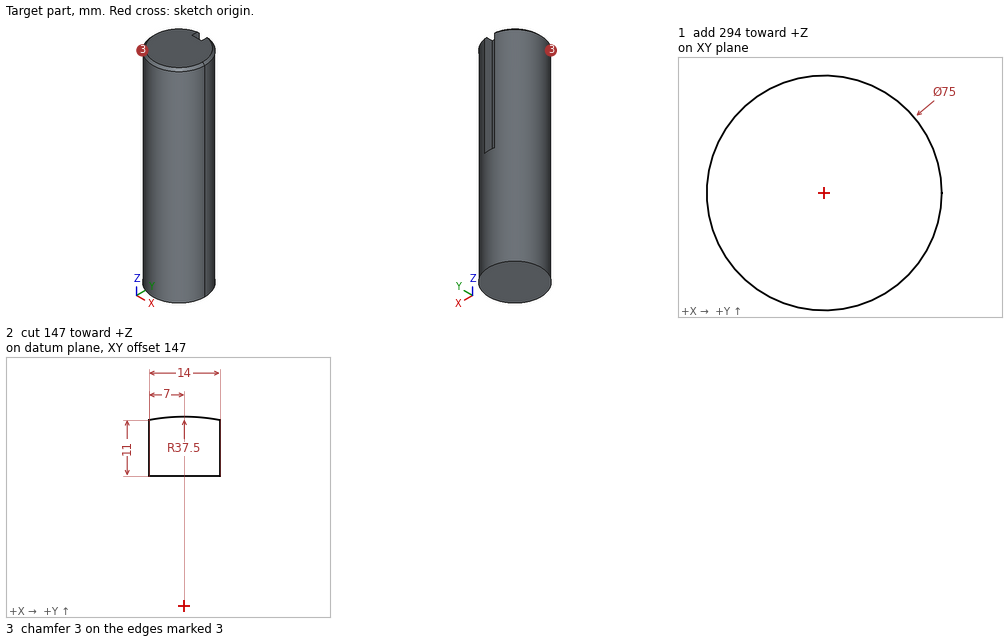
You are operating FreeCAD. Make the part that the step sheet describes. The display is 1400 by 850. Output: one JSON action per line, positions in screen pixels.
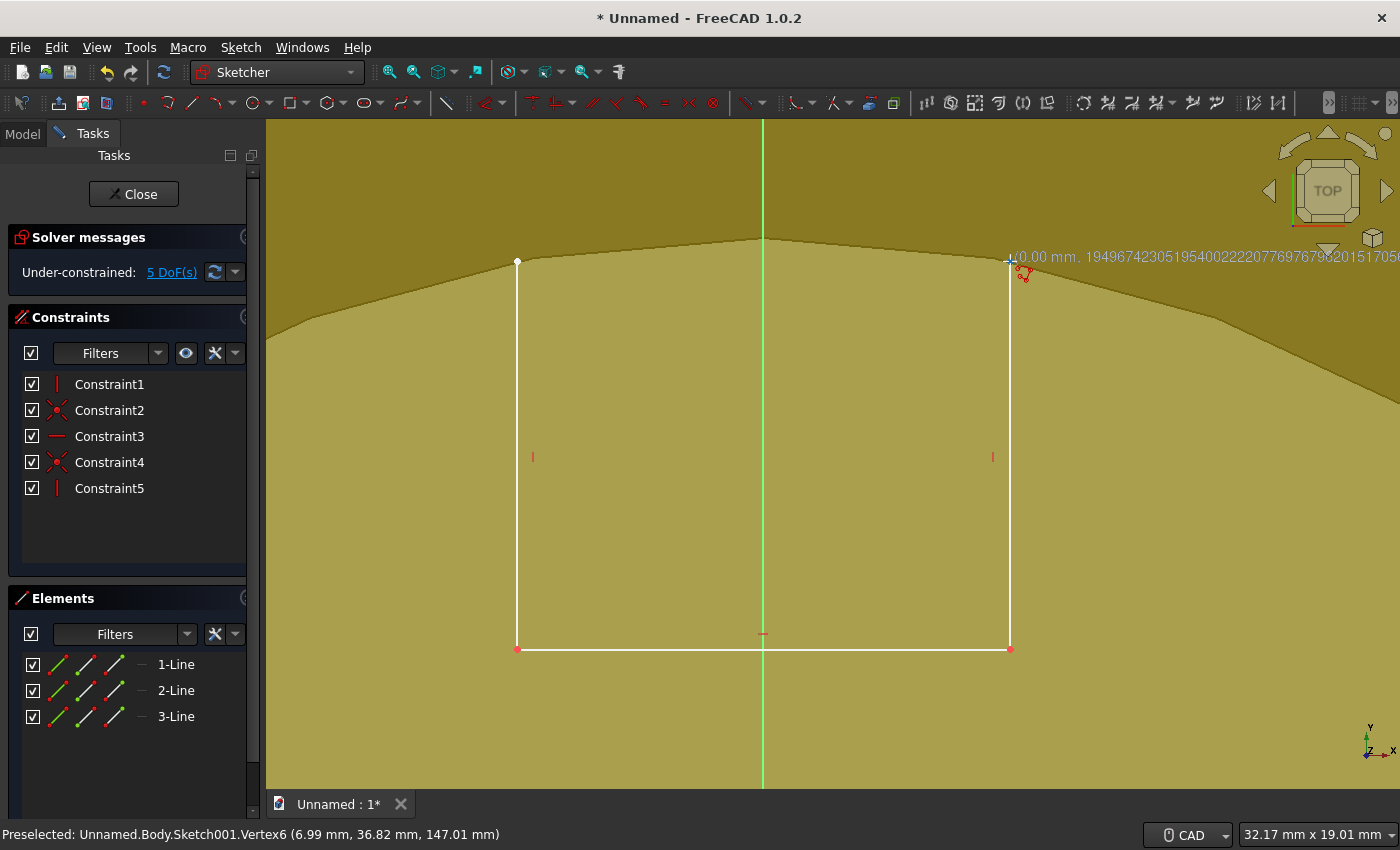
{"action": "left_click", "coordinate": [216, 104]}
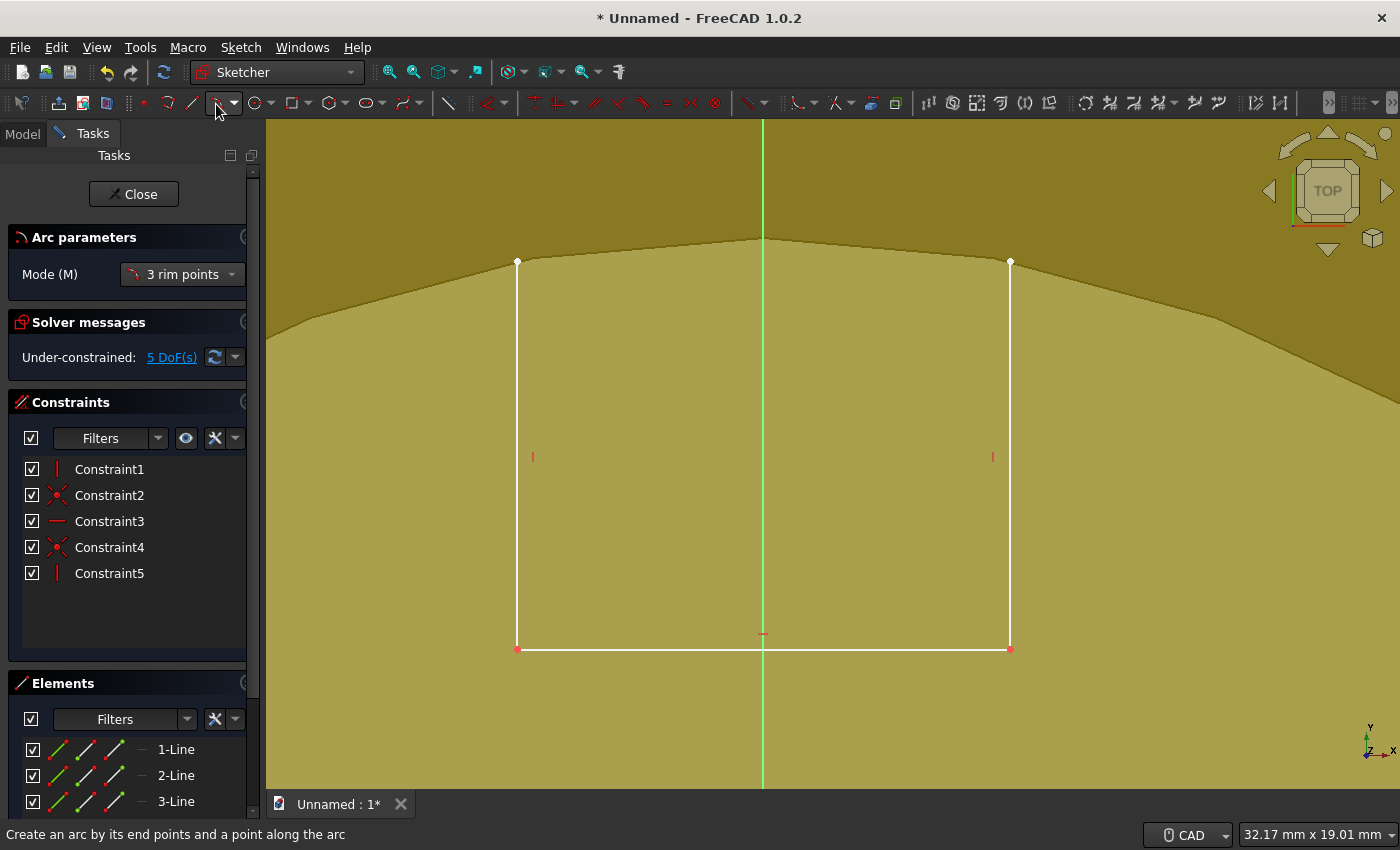
{"action": "left_click", "coordinate": [1010, 262]}
{"action": "left_click", "coordinate": [517, 262]}
{"action": "left_click", "coordinate": [813, 239]}
{"action": "key", "text": "Escape"}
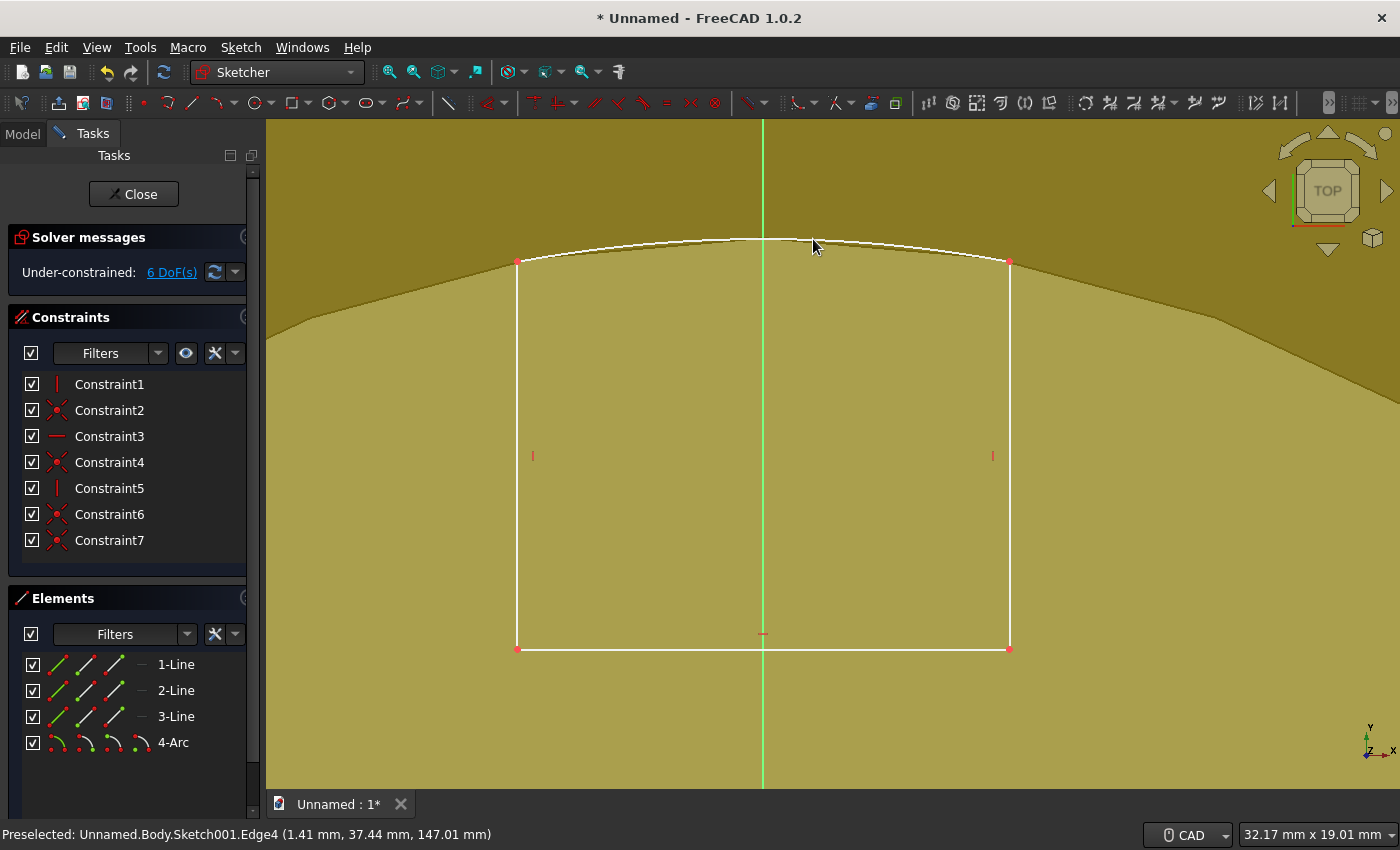
{"action": "scroll", "coordinate": [765, 260], "scroll_direction": "down", "scroll_amount": 6}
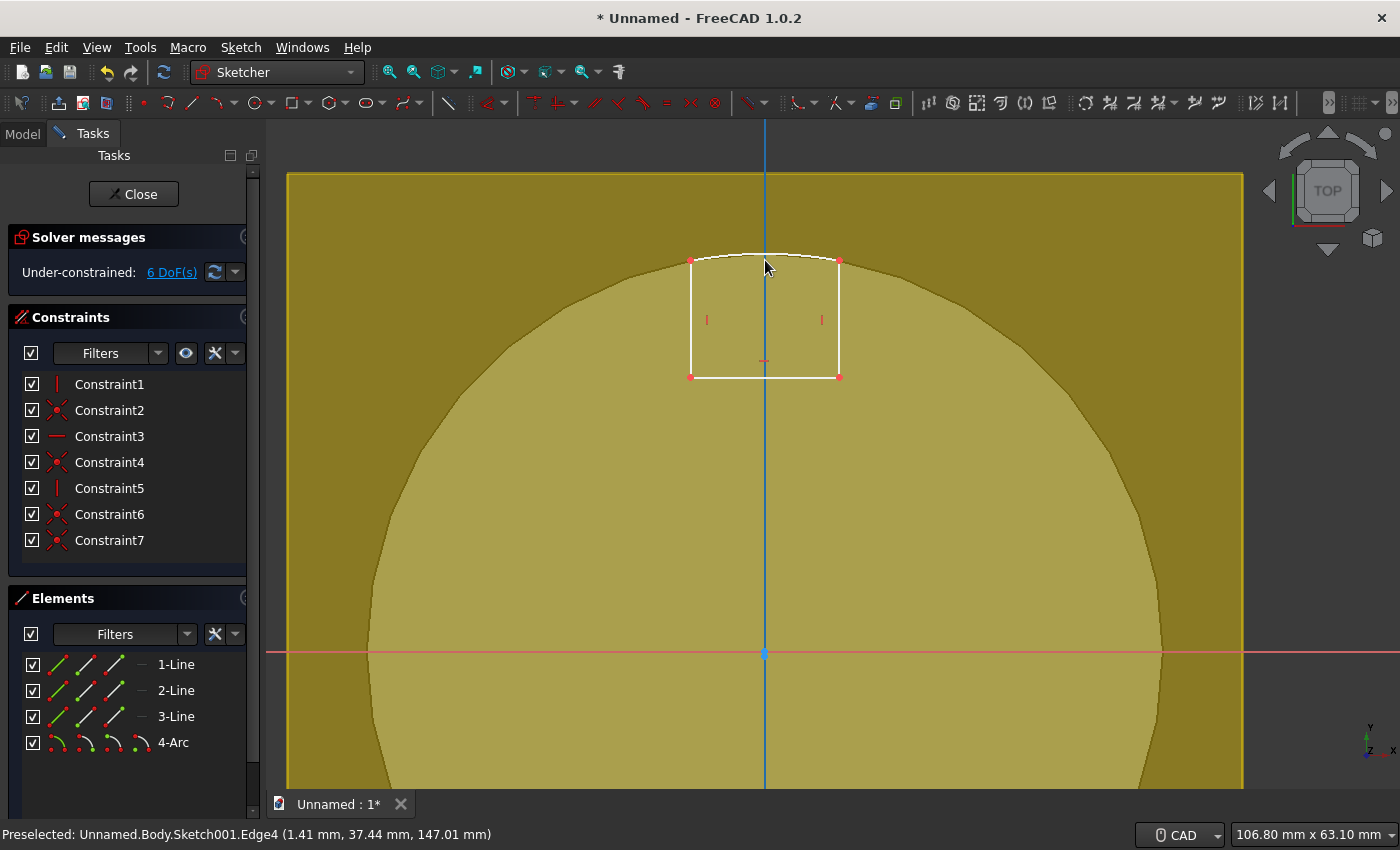
{"action": "left_click_drag", "start_coordinate": [755, 642], "coordinate": [775, 667]}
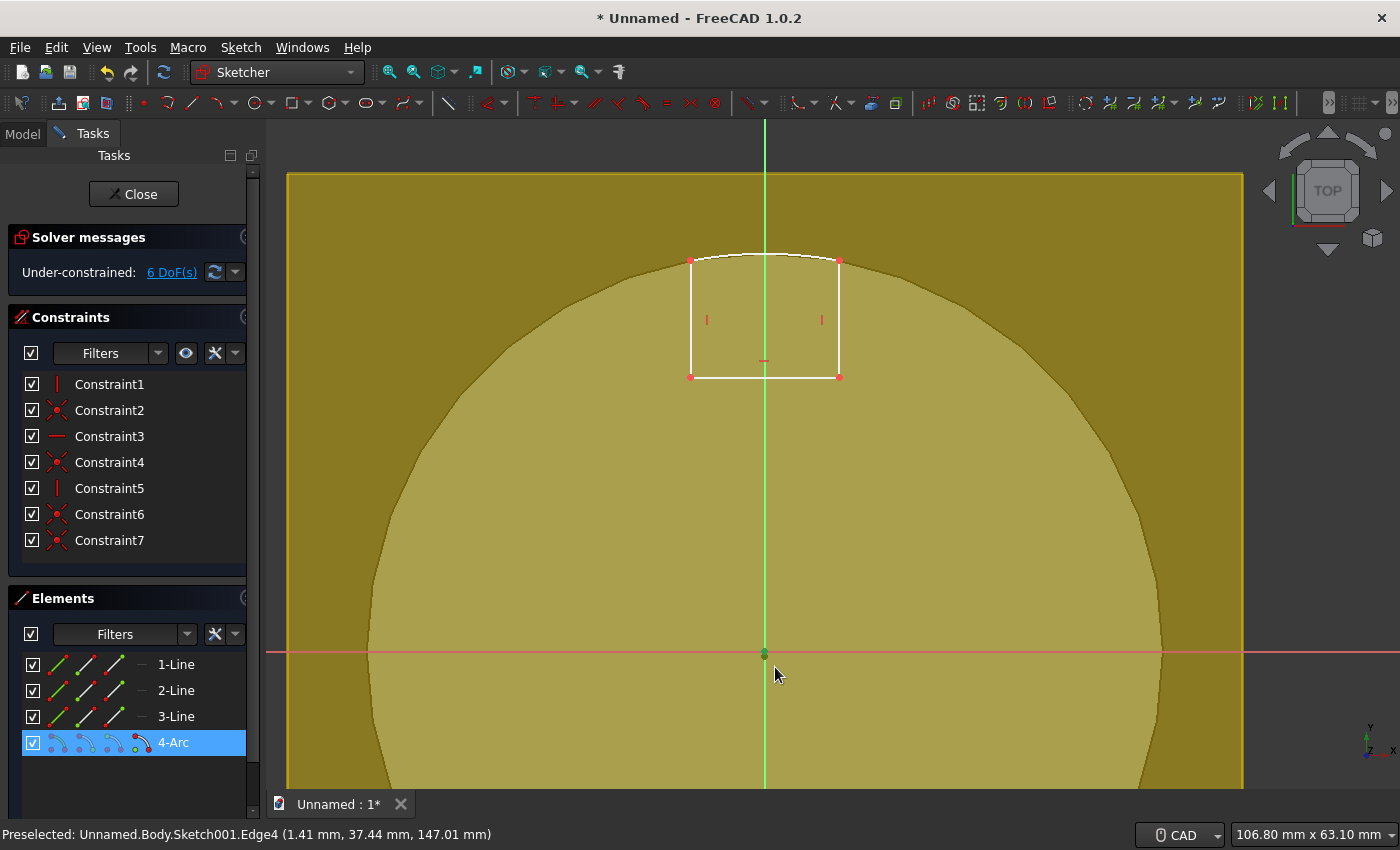
{"action": "key", "text": "c"}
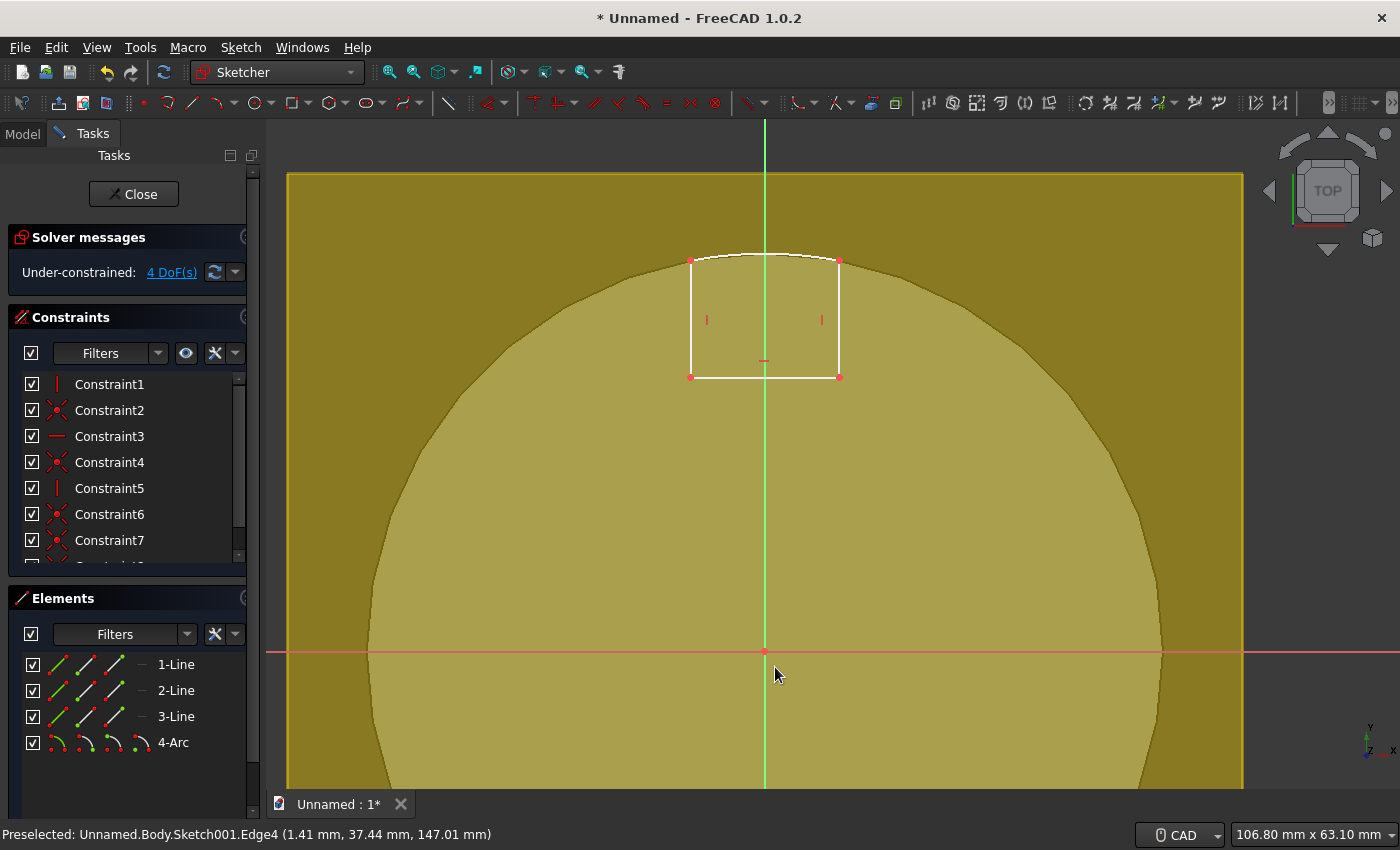
{"action": "left_click", "coordinate": [488, 104]}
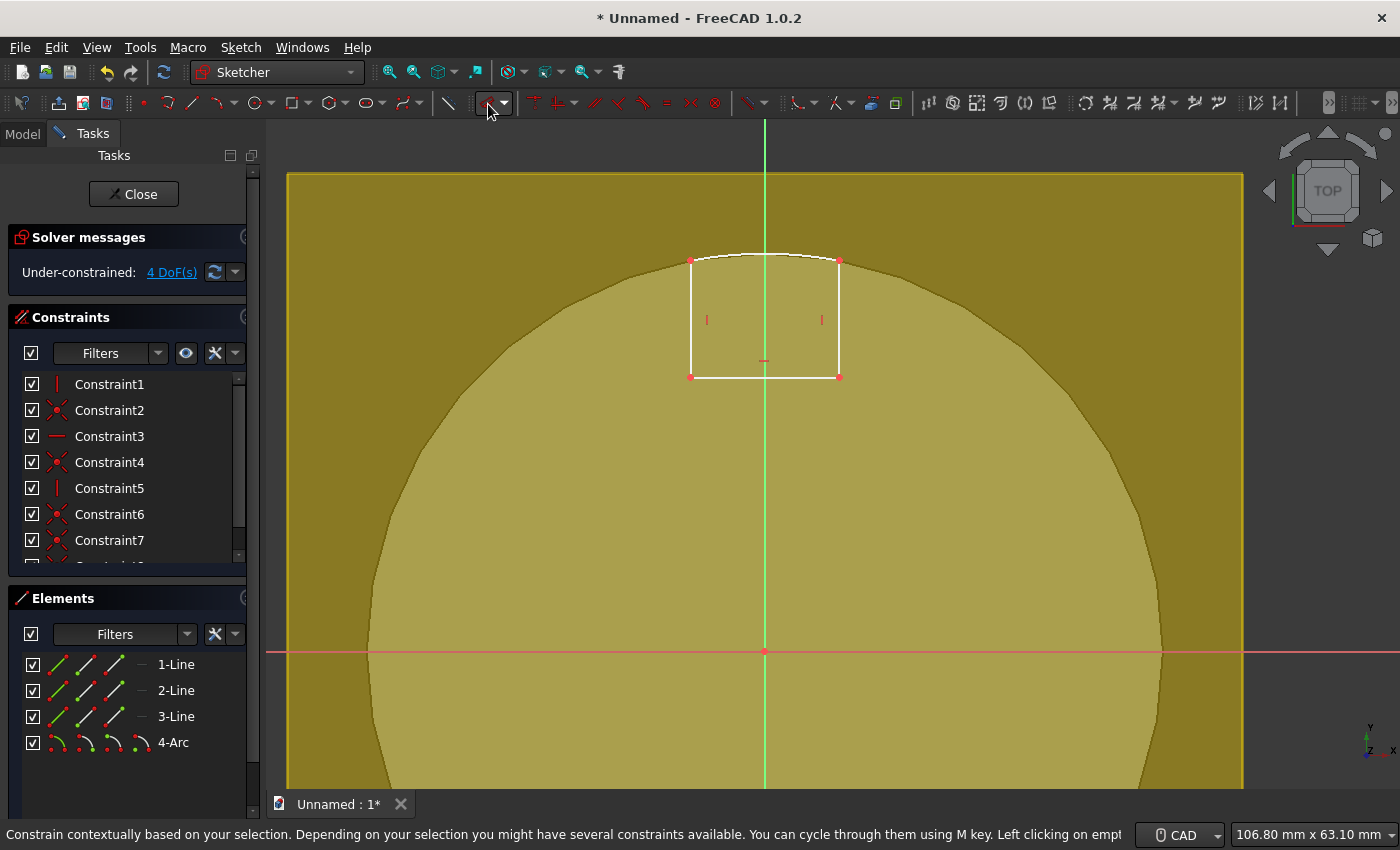
{"action": "left_click", "coordinate": [795, 255]}
{"action": "left_click", "coordinate": [797, 223]}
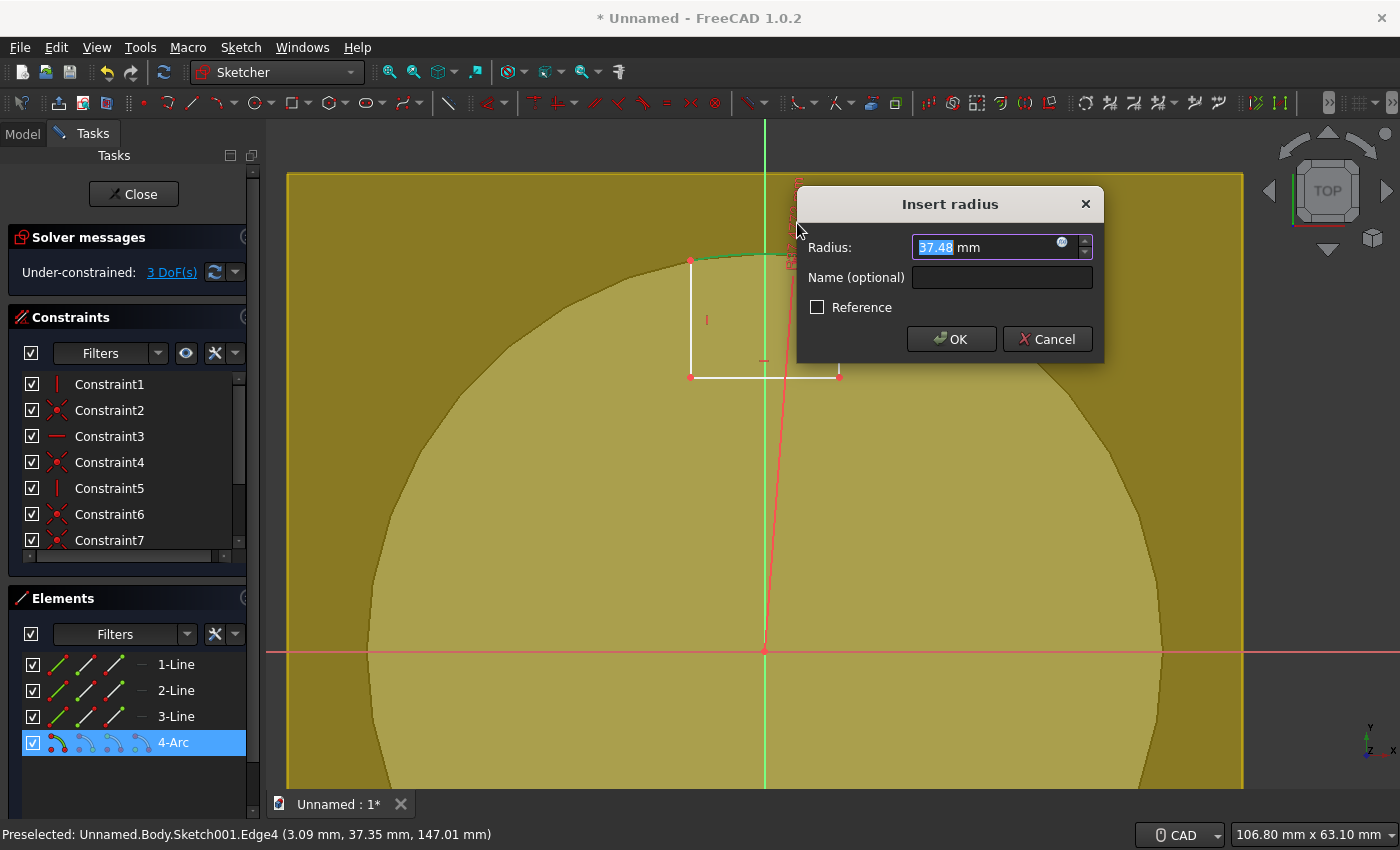
{"action": "type", "text": "37.5"}
{"action": "key", "text": "Return"}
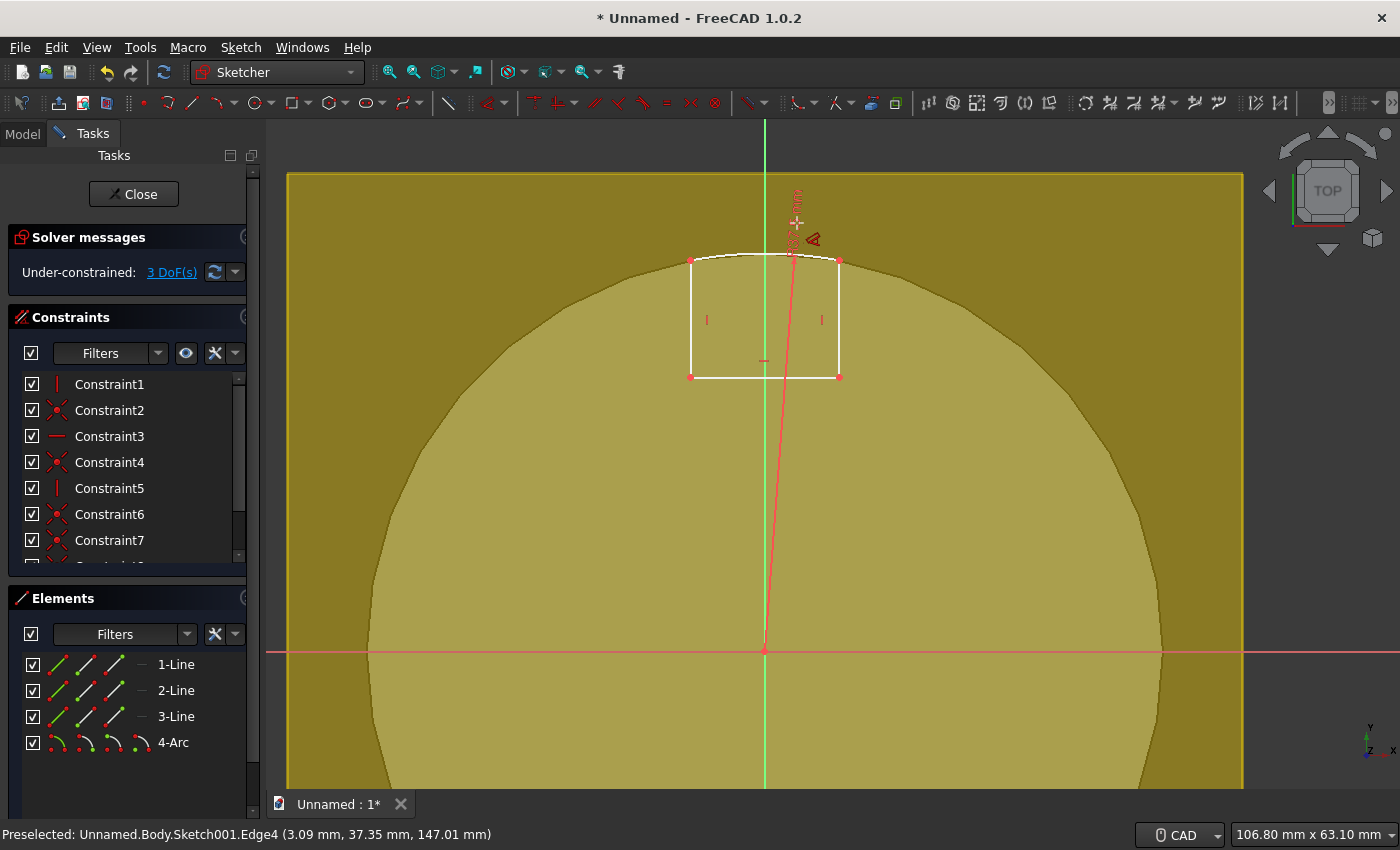
{"action": "left_click", "coordinate": [691, 296]}
{"action": "left_click", "coordinate": [657, 319]}